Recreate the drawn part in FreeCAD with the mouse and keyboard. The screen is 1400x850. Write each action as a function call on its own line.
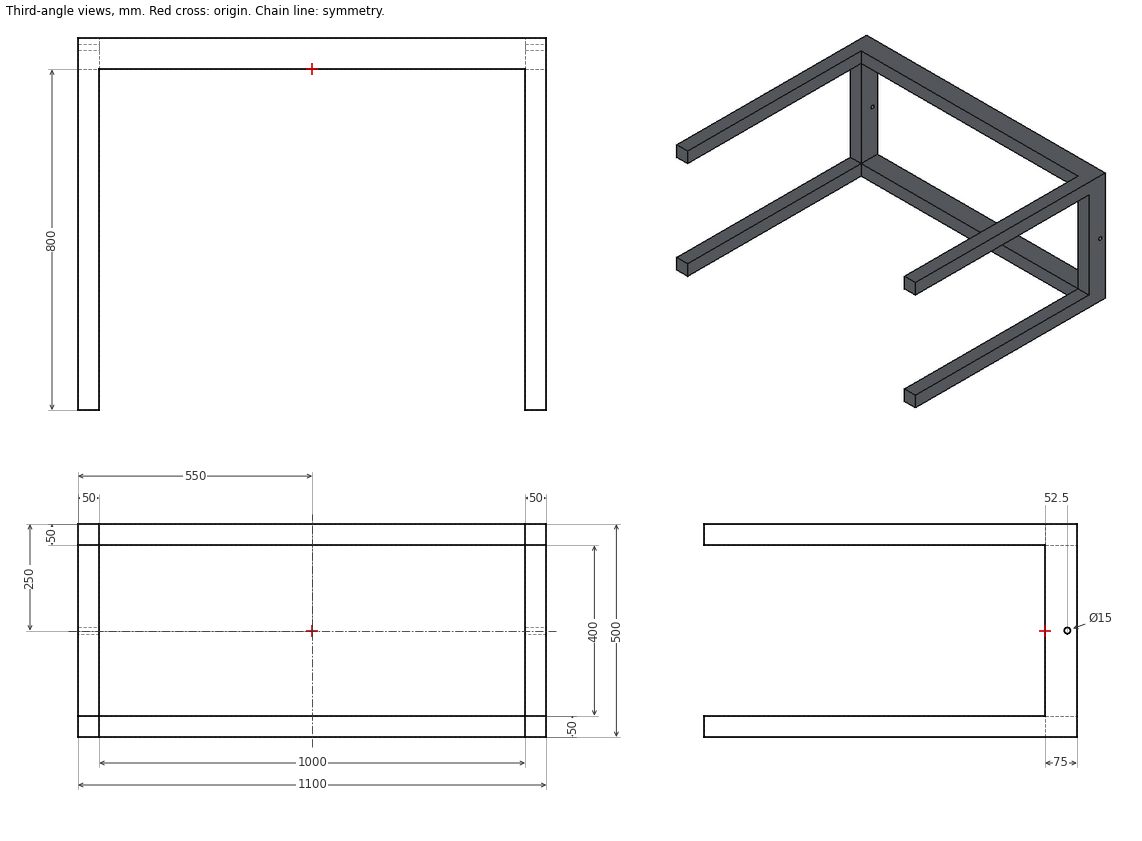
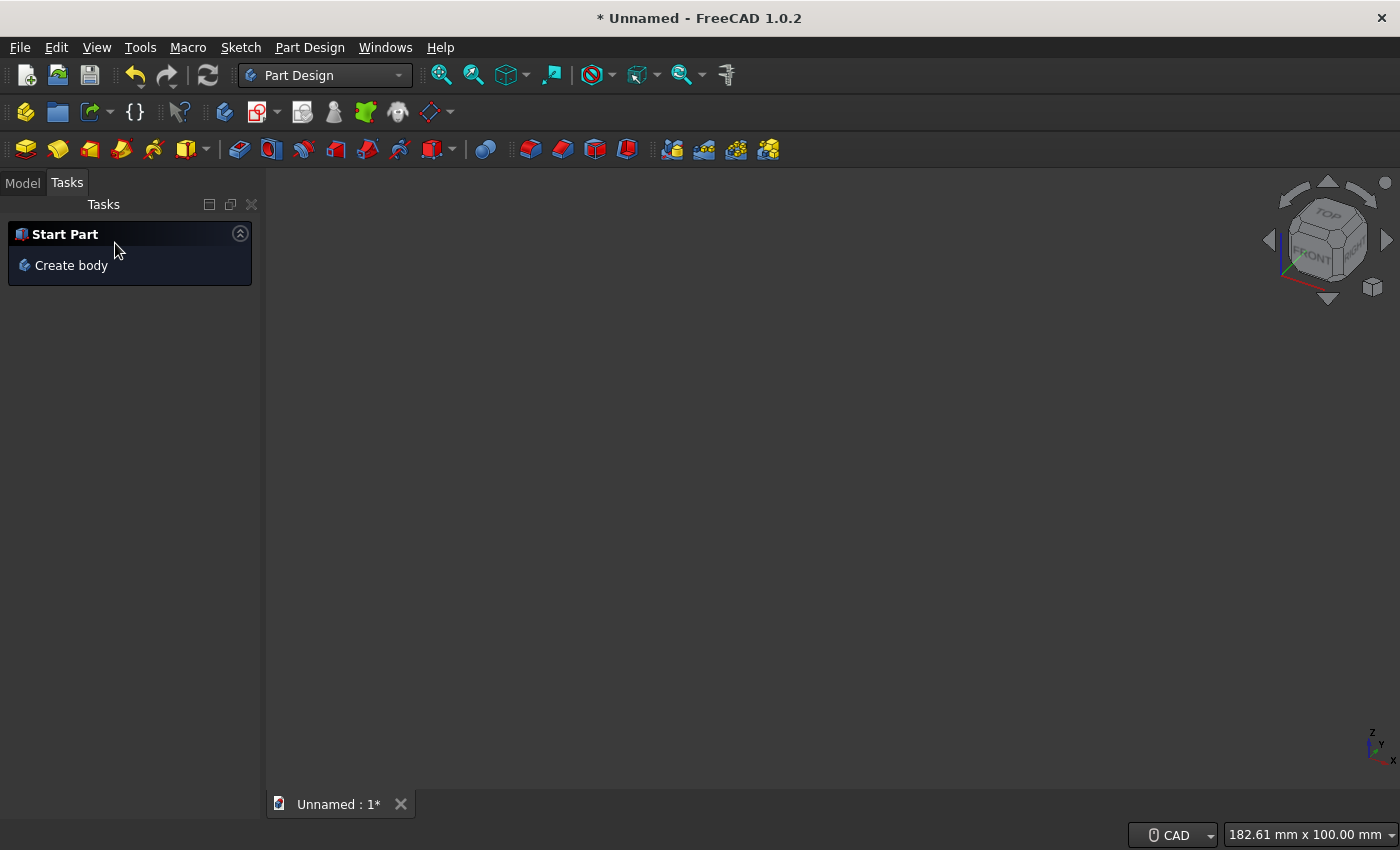
click(442, 76)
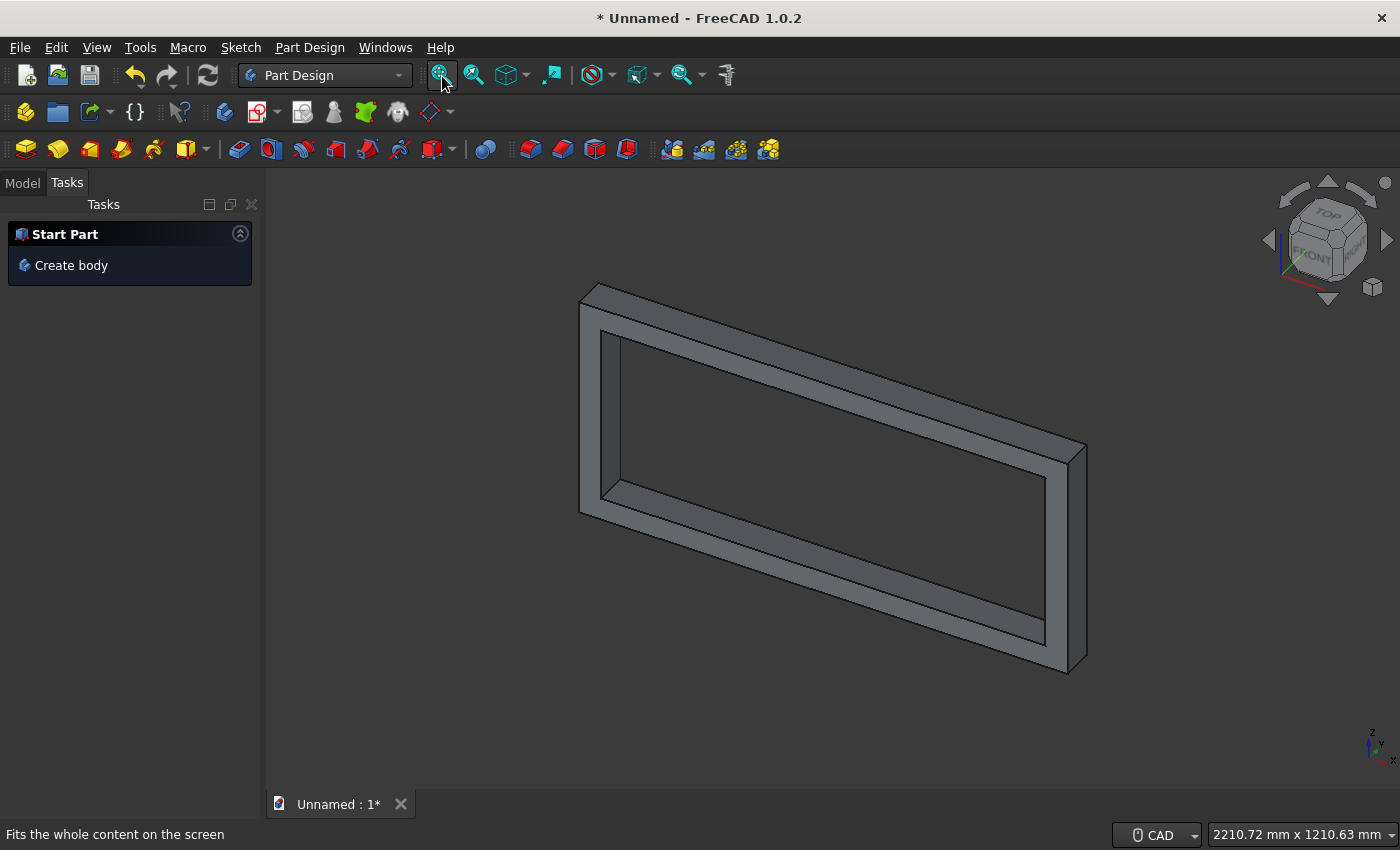
click(1033, 466)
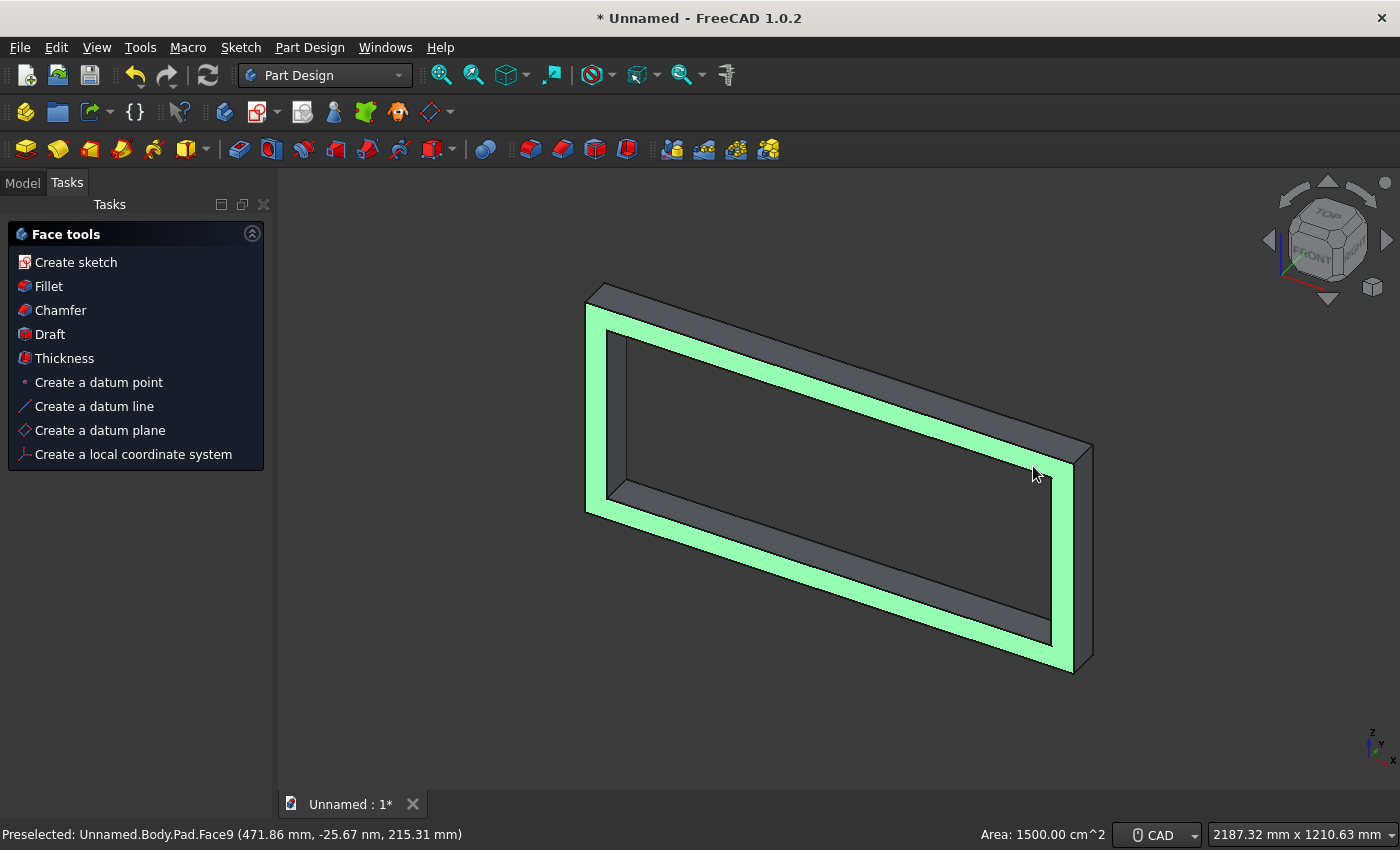
click(258, 112)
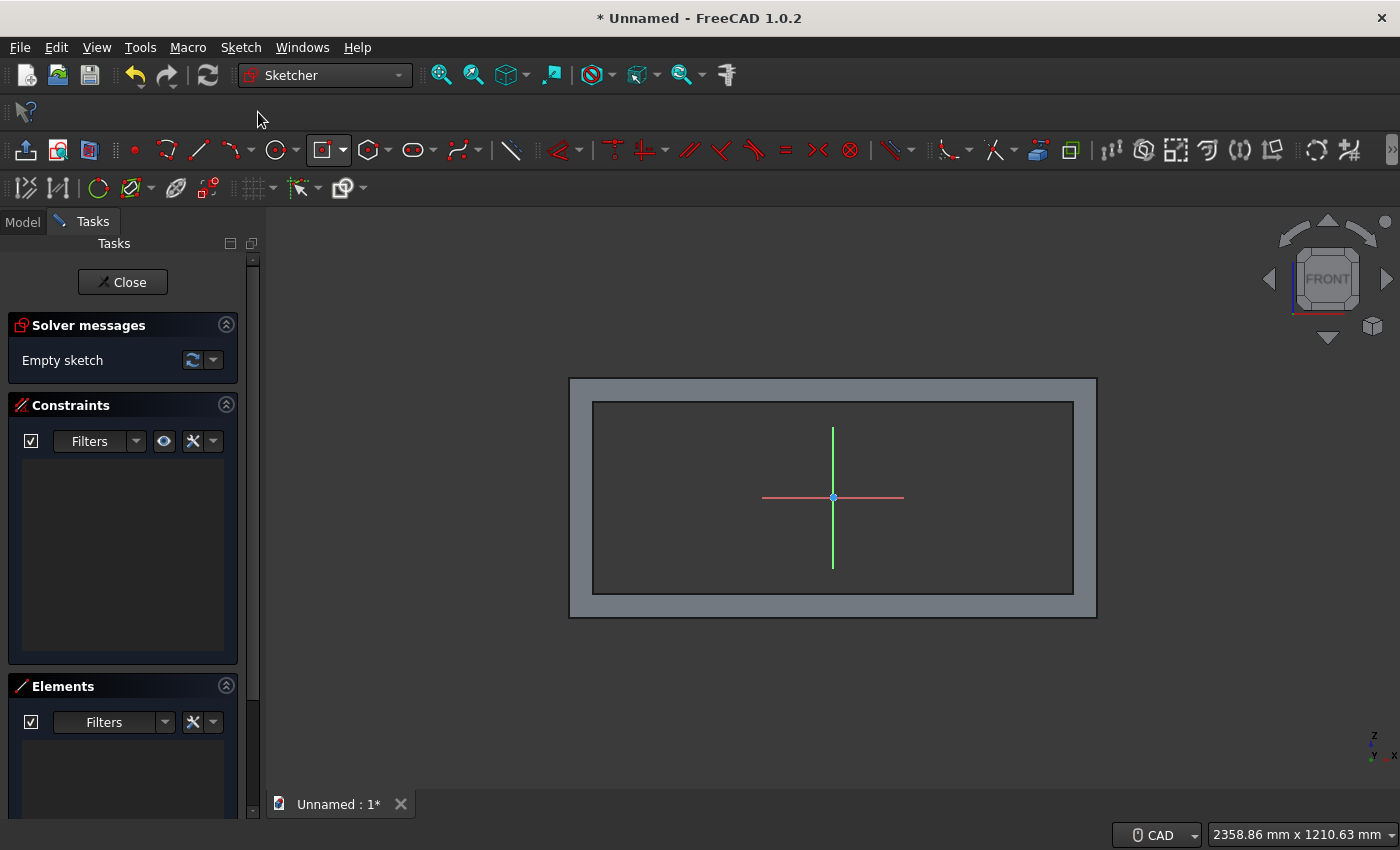
key(g)
key(r)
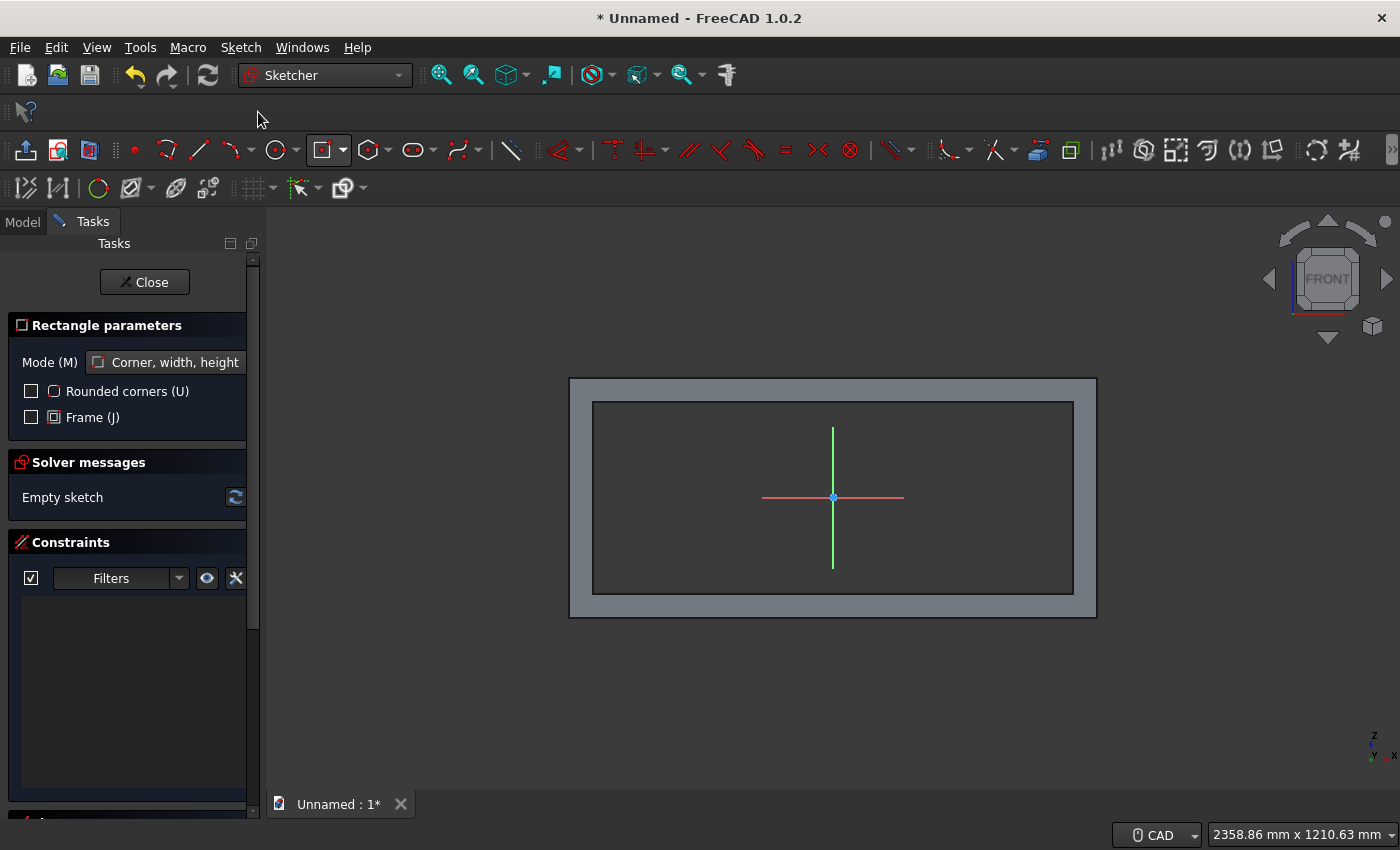
click(569, 378)
move(593, 402)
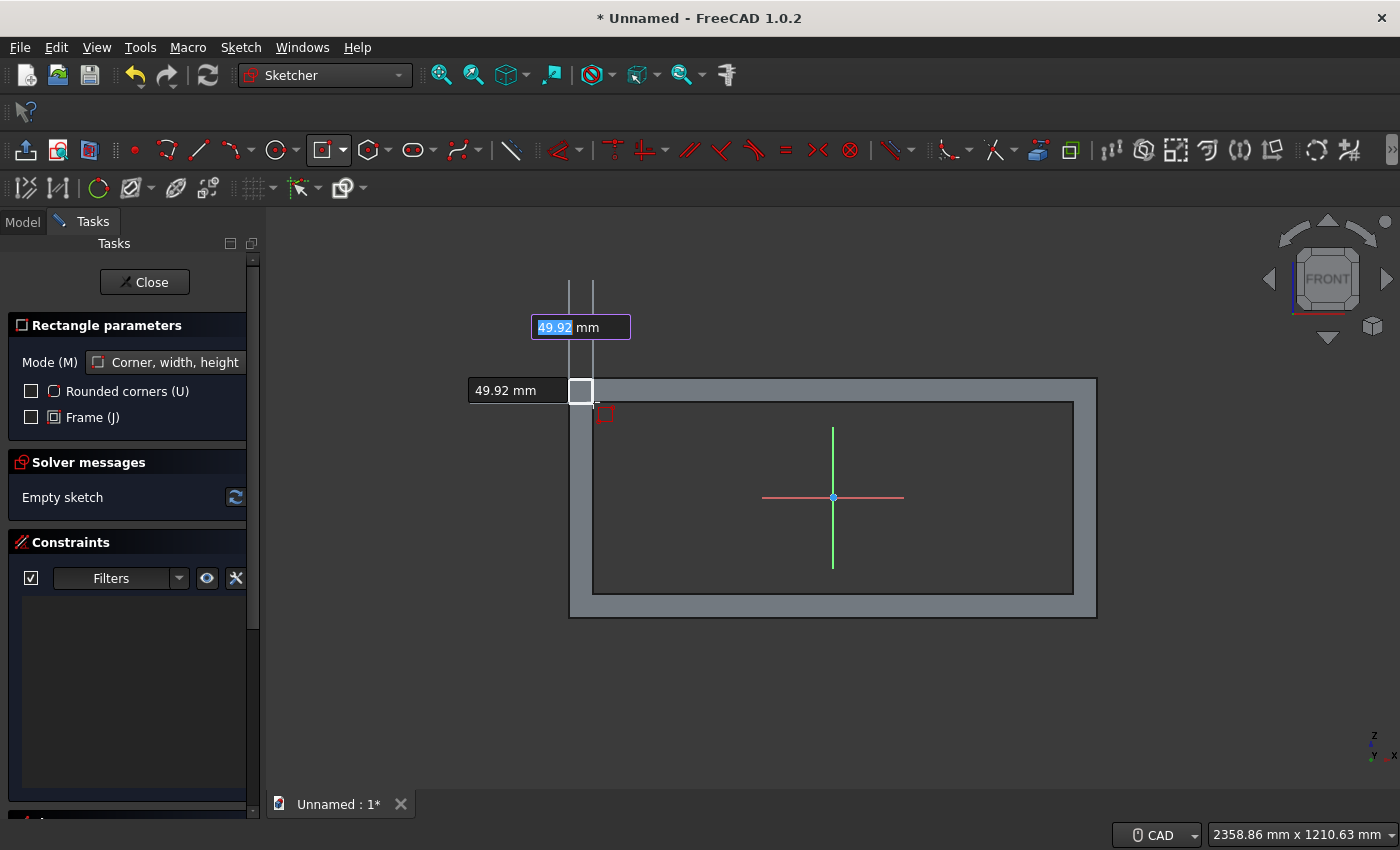
text(50)
key(Tab)
text(50)
key(Return)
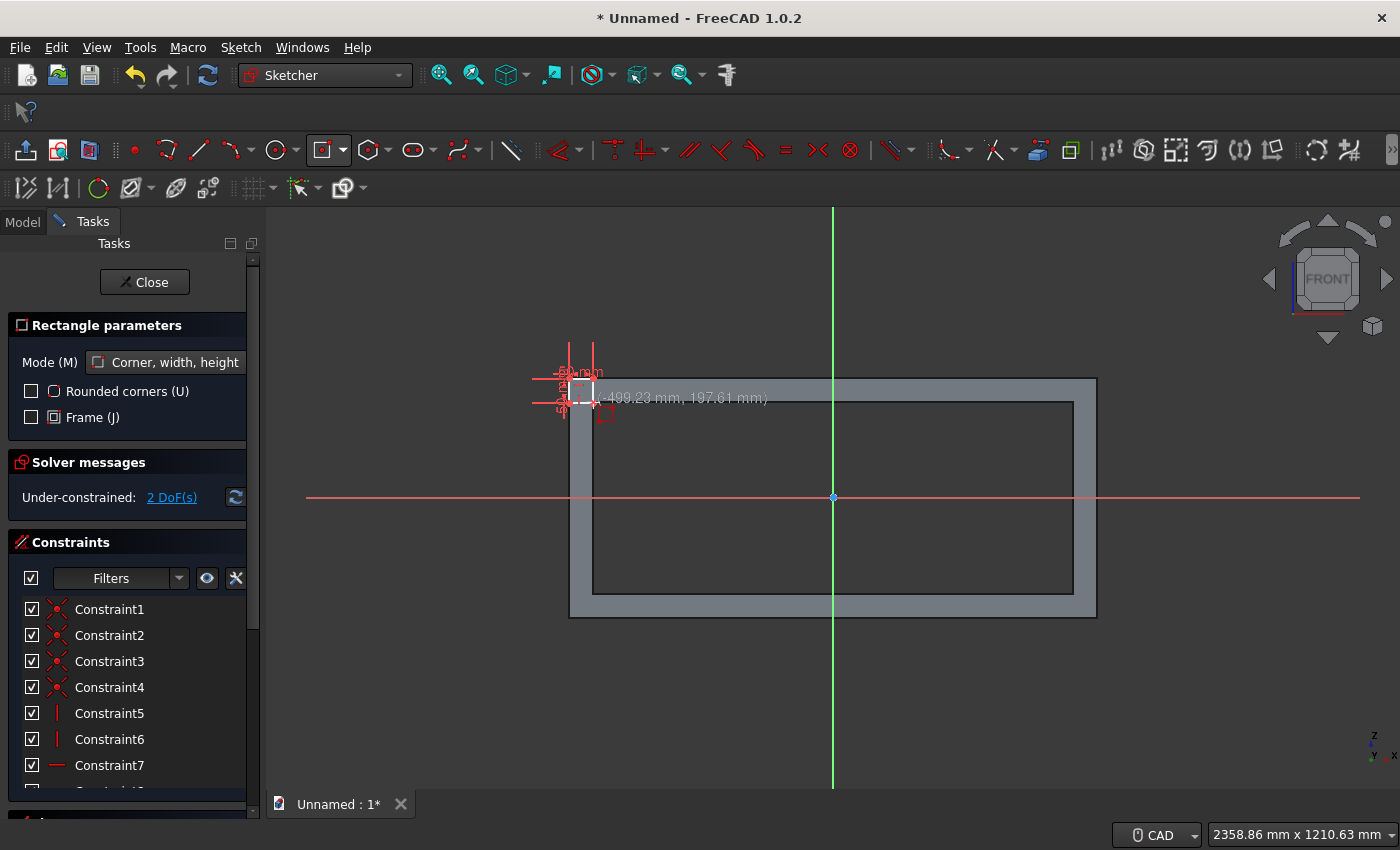
click(1073, 378)
move(1097, 402)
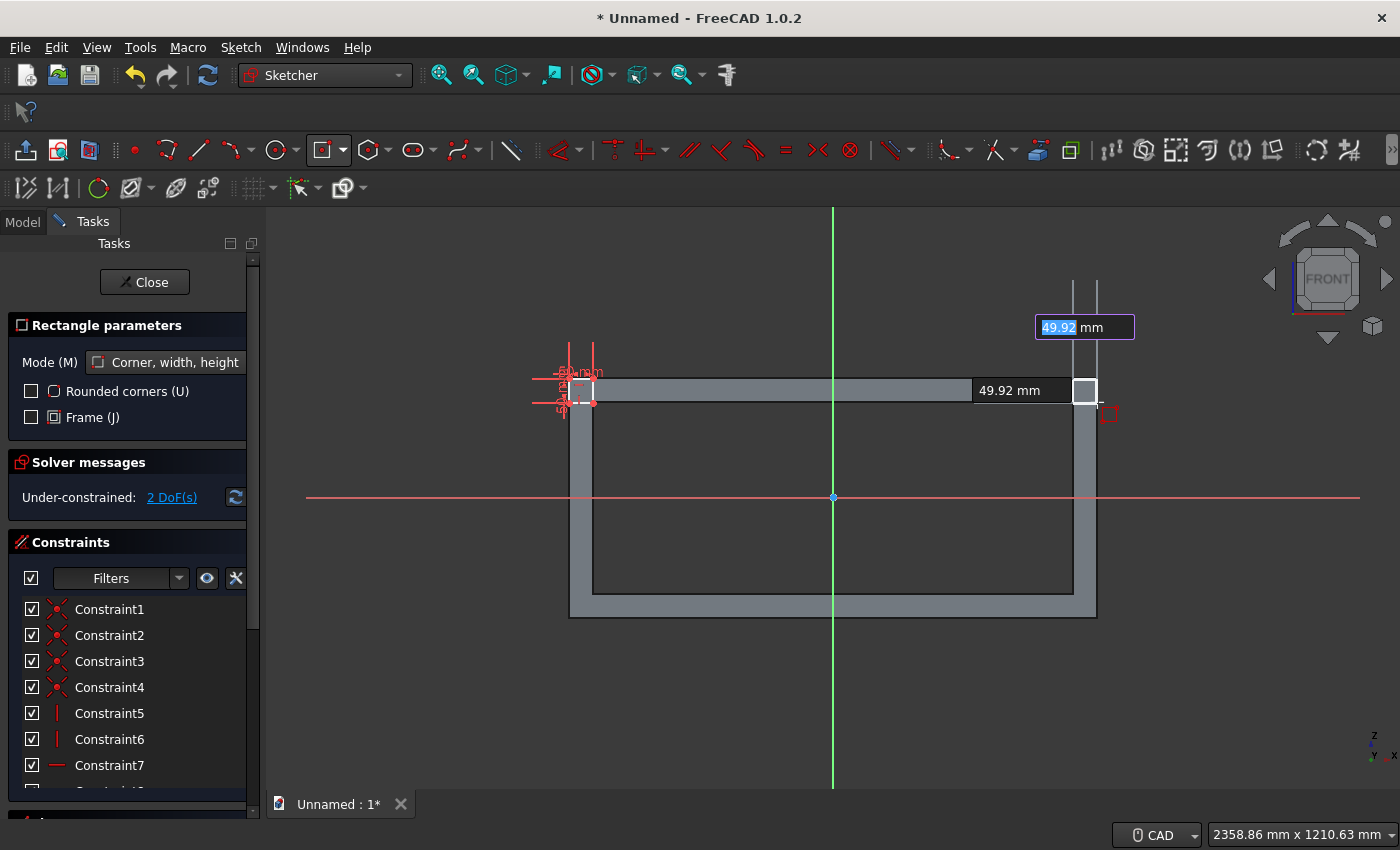
text(50)
key(Tab)
text(50)
key(Return)